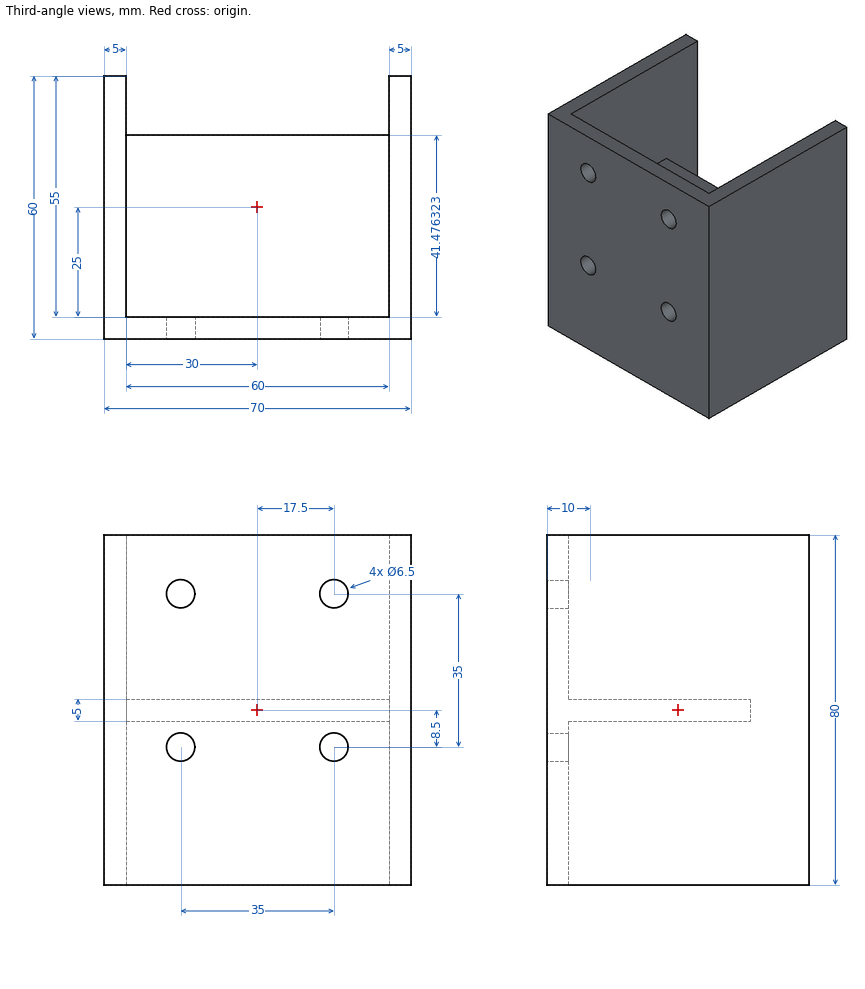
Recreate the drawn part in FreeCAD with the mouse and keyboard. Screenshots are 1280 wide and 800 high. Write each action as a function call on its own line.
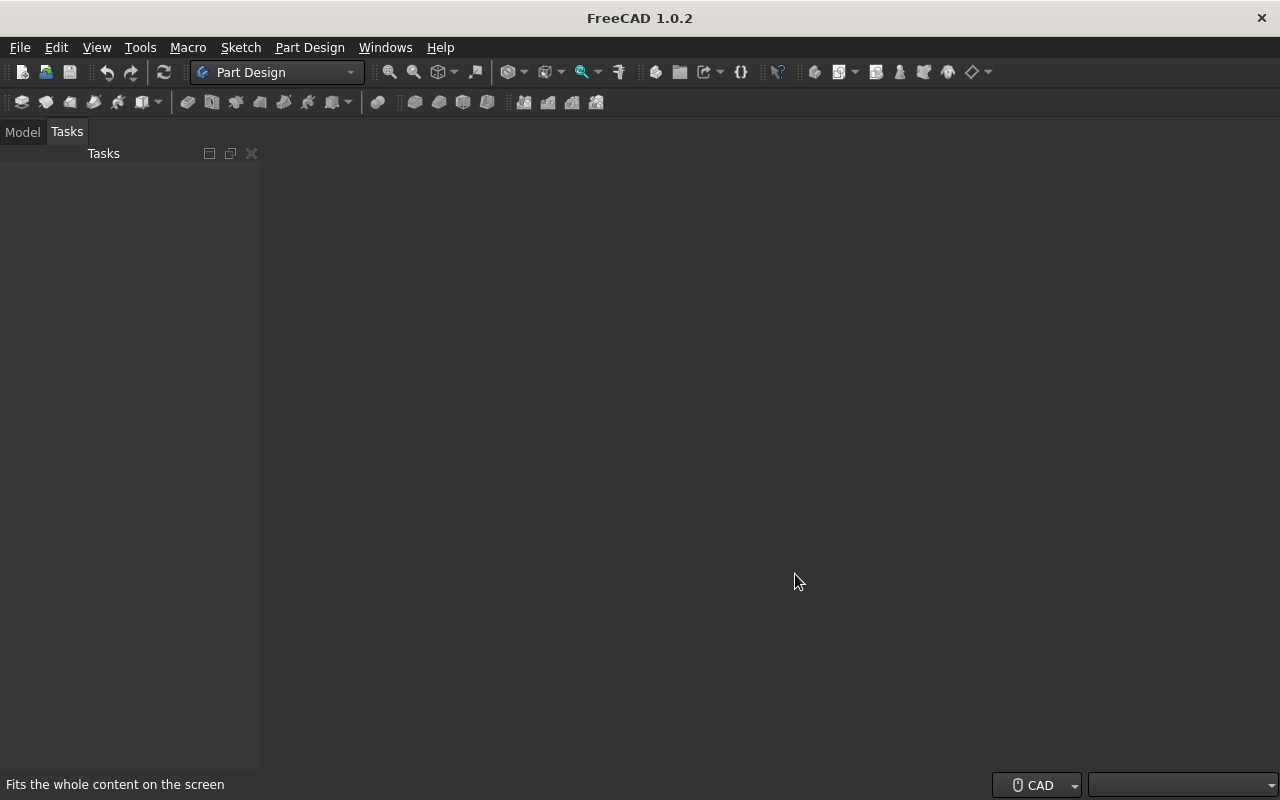
key(ctrl+n)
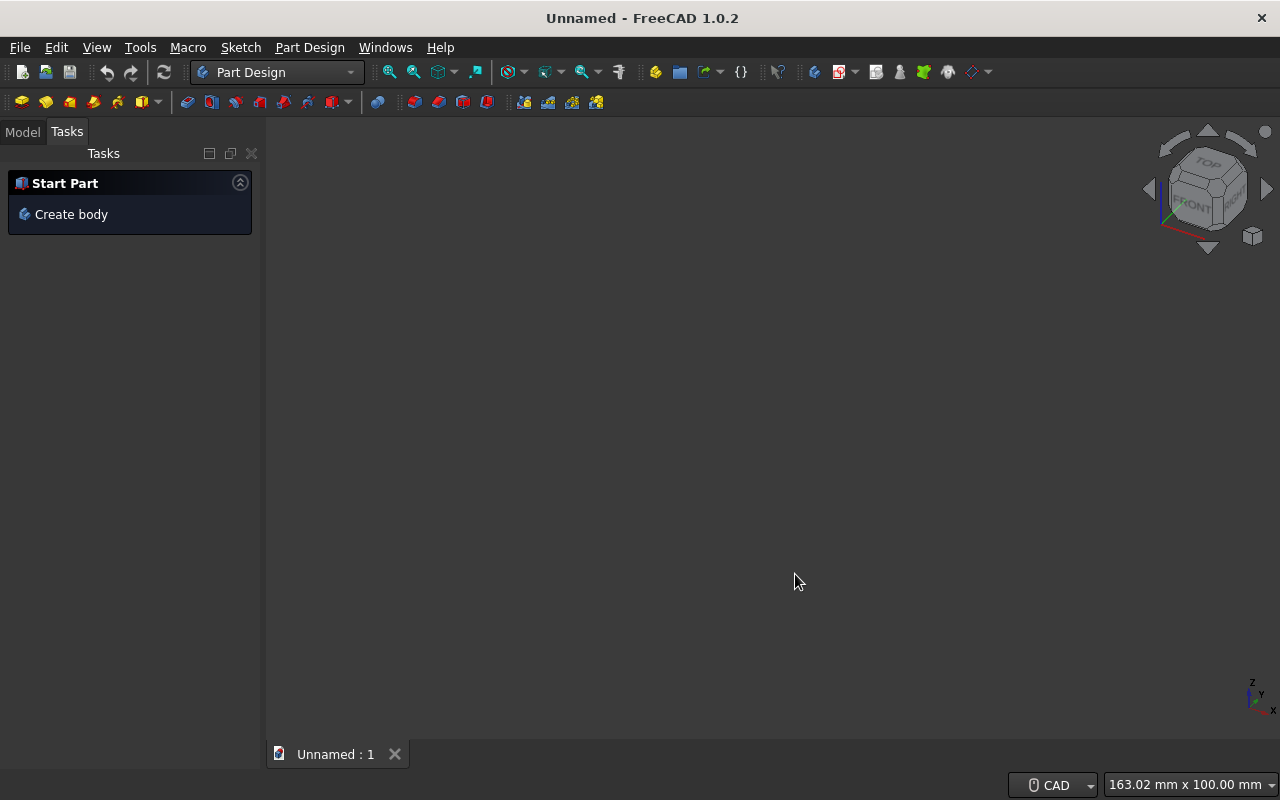
click(840, 72)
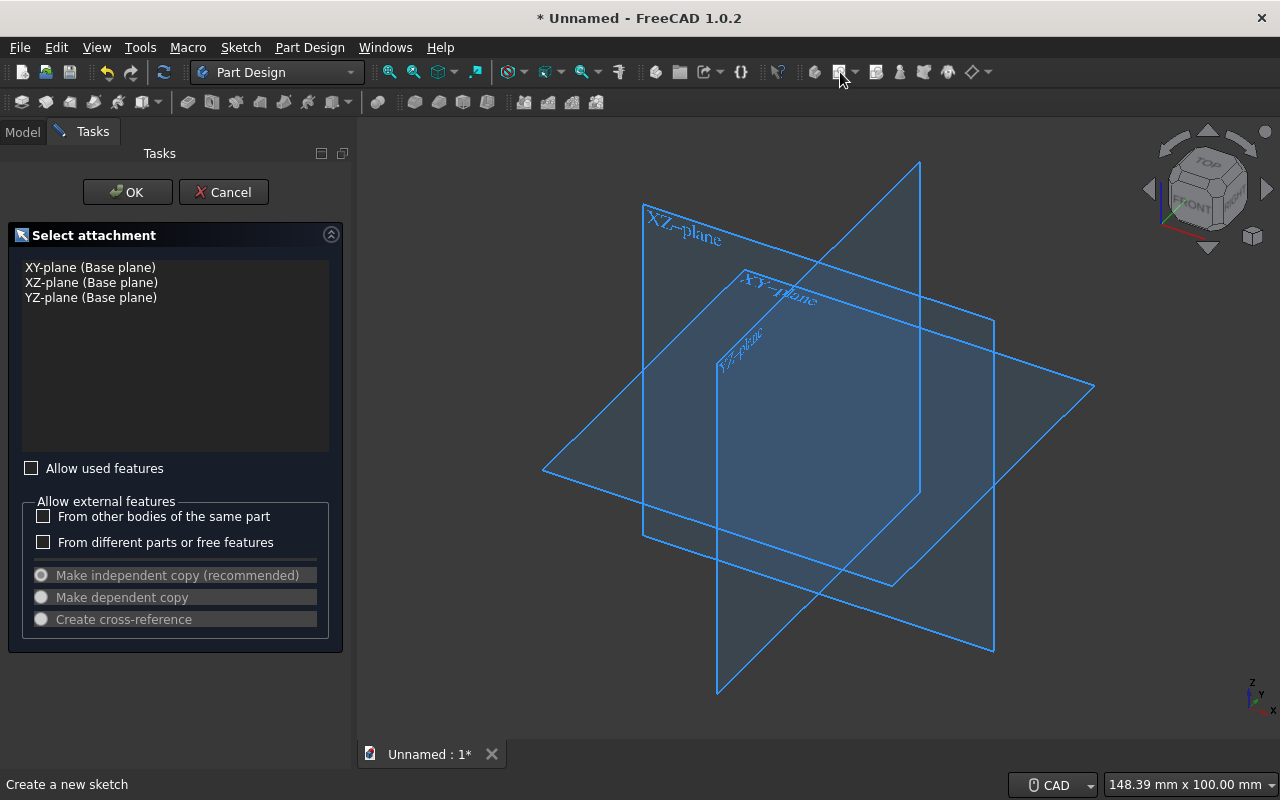
click(82, 268)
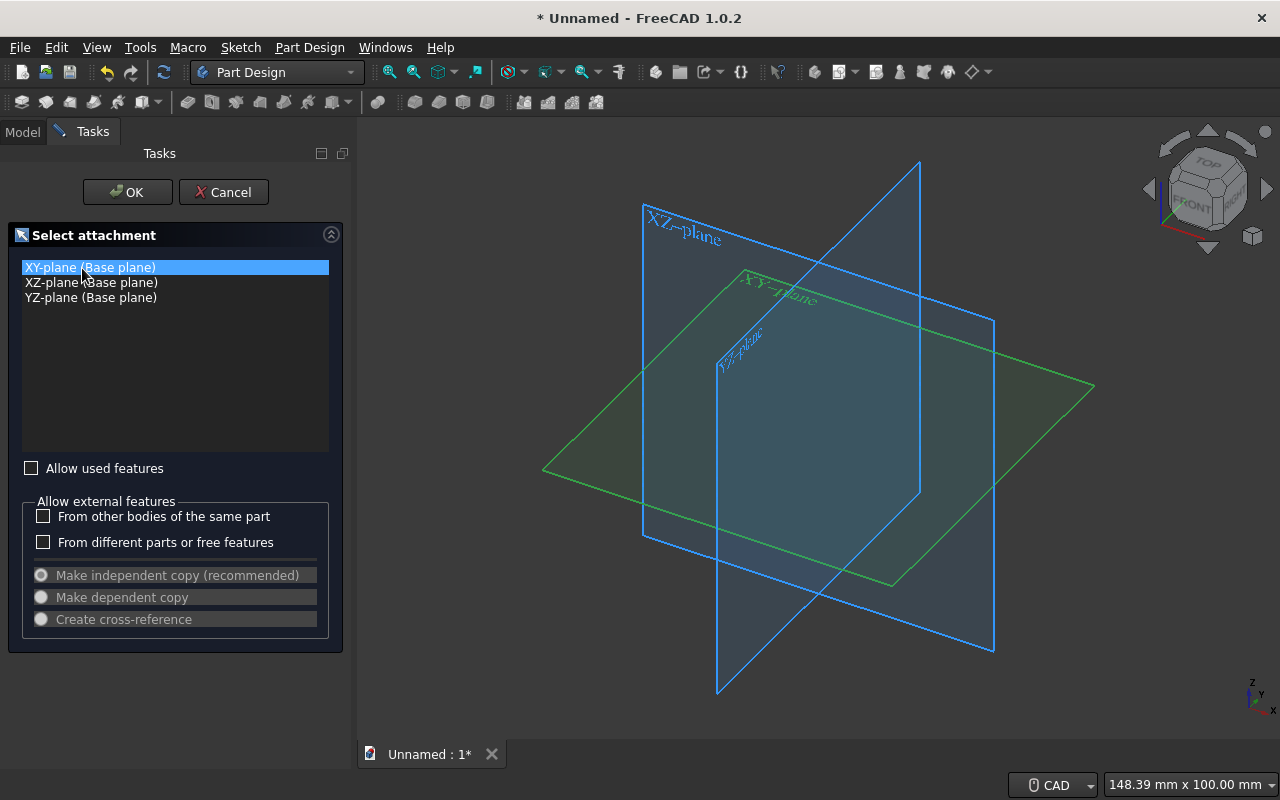
click(128, 192)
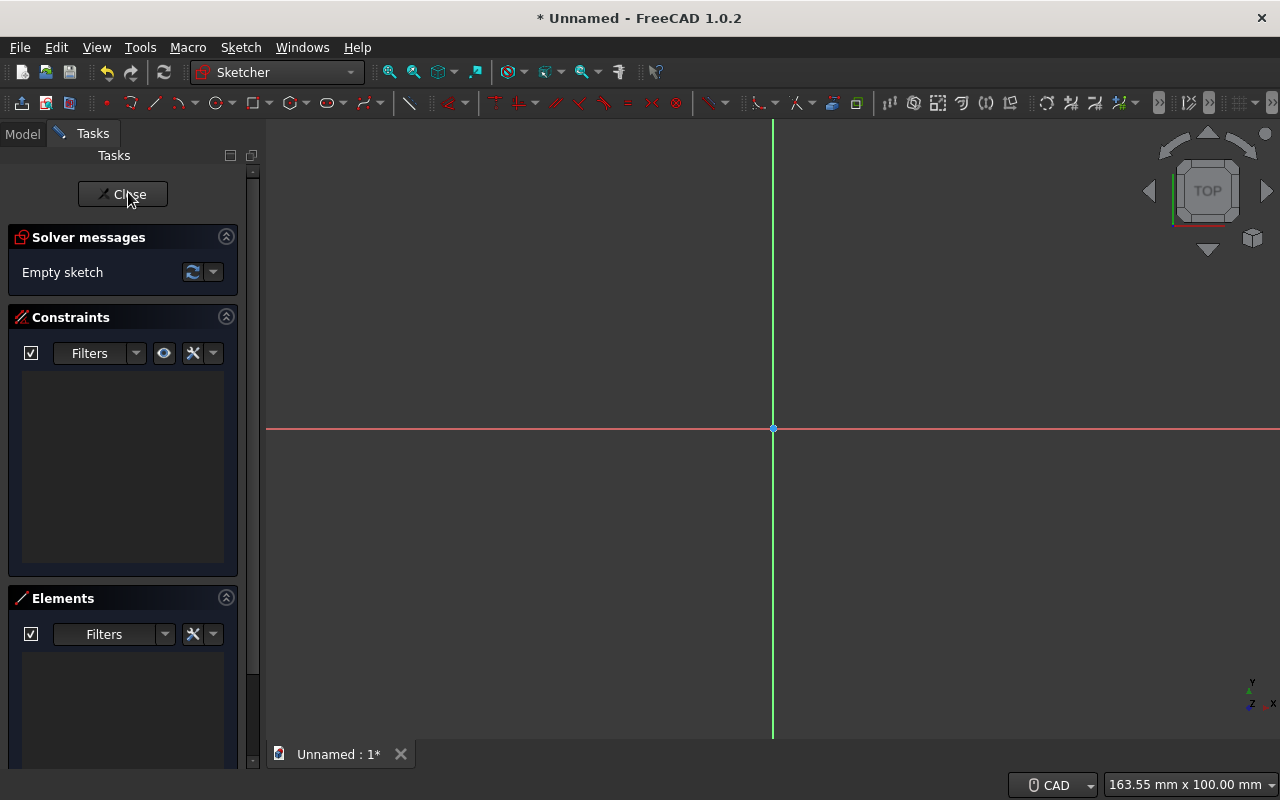
key(g)
key(m)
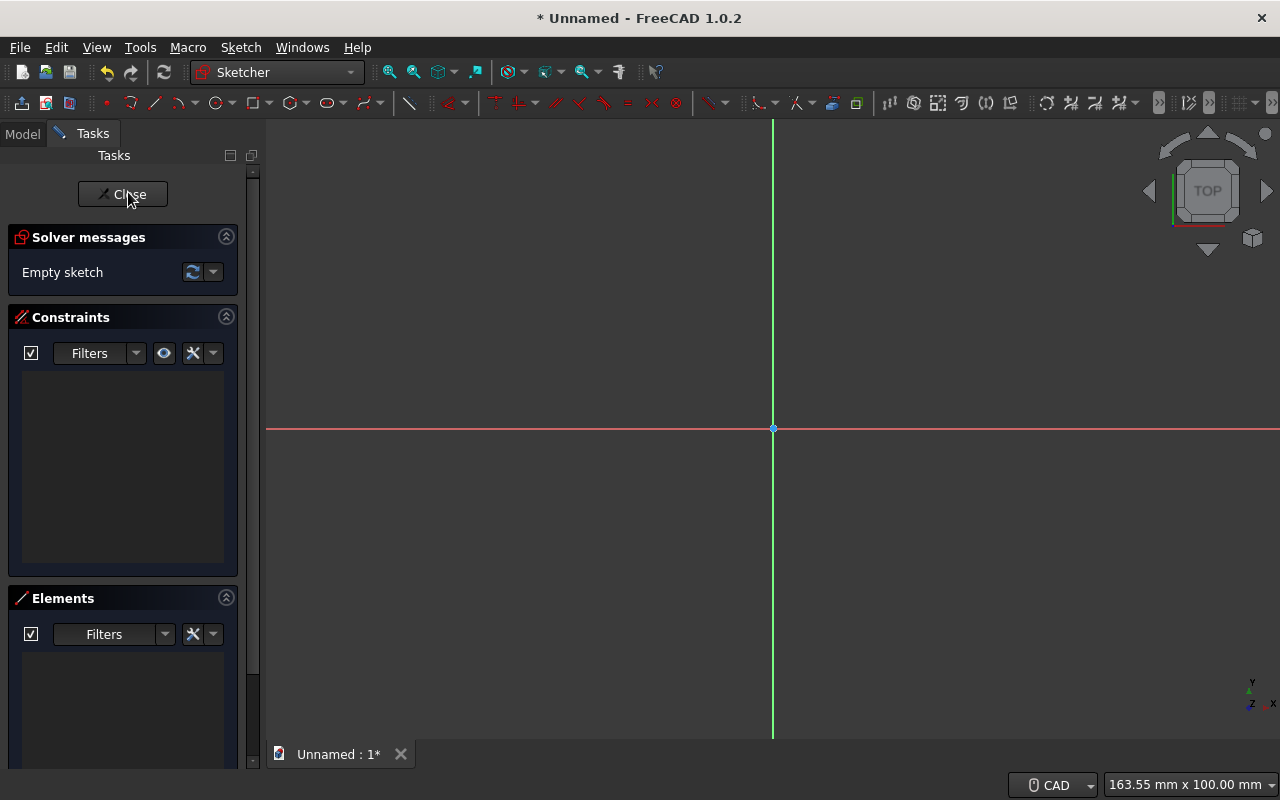
click(587, 584)
click(587, 243)
click(556, 243)
click(556, 615)
click(990, 615)
click(990, 243)
click(959, 243)
click(959, 584)
click(587, 585)
key(Escape)
key(Escape)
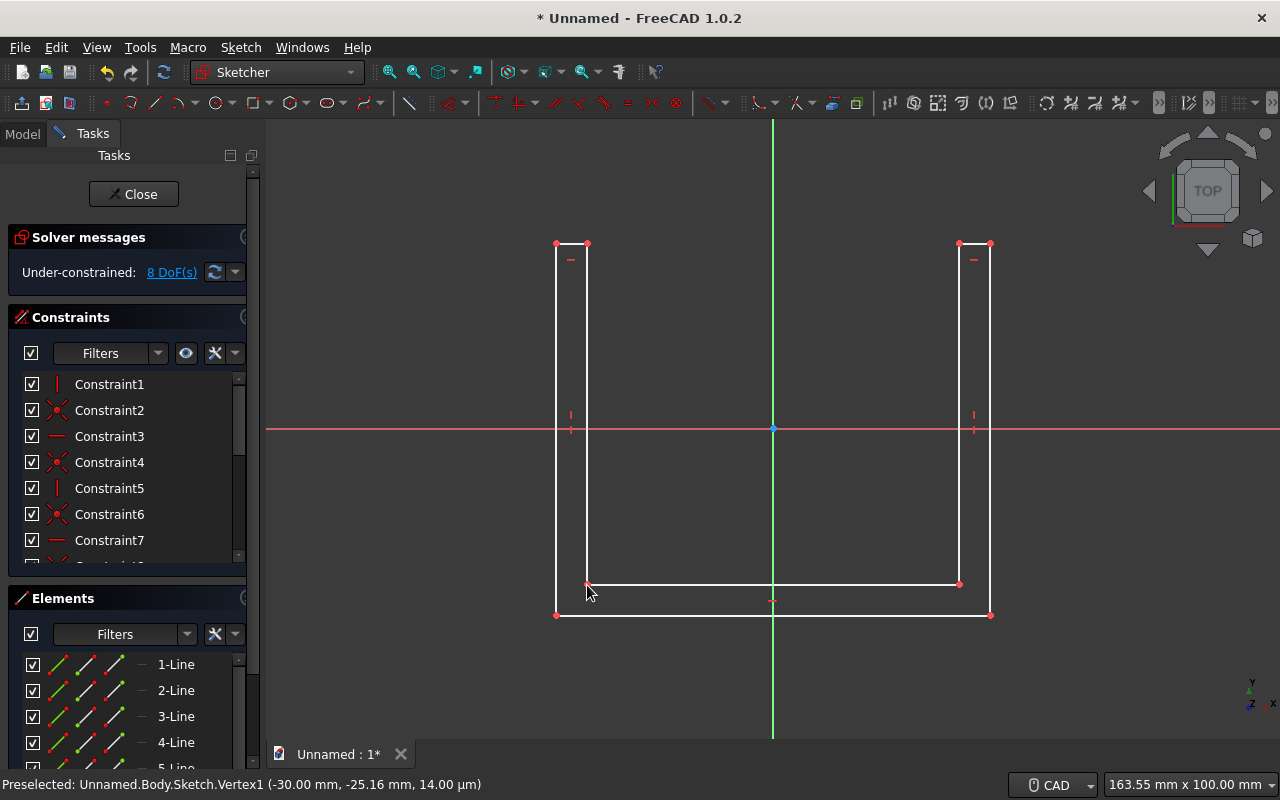
scroll(578, 244, up, 2)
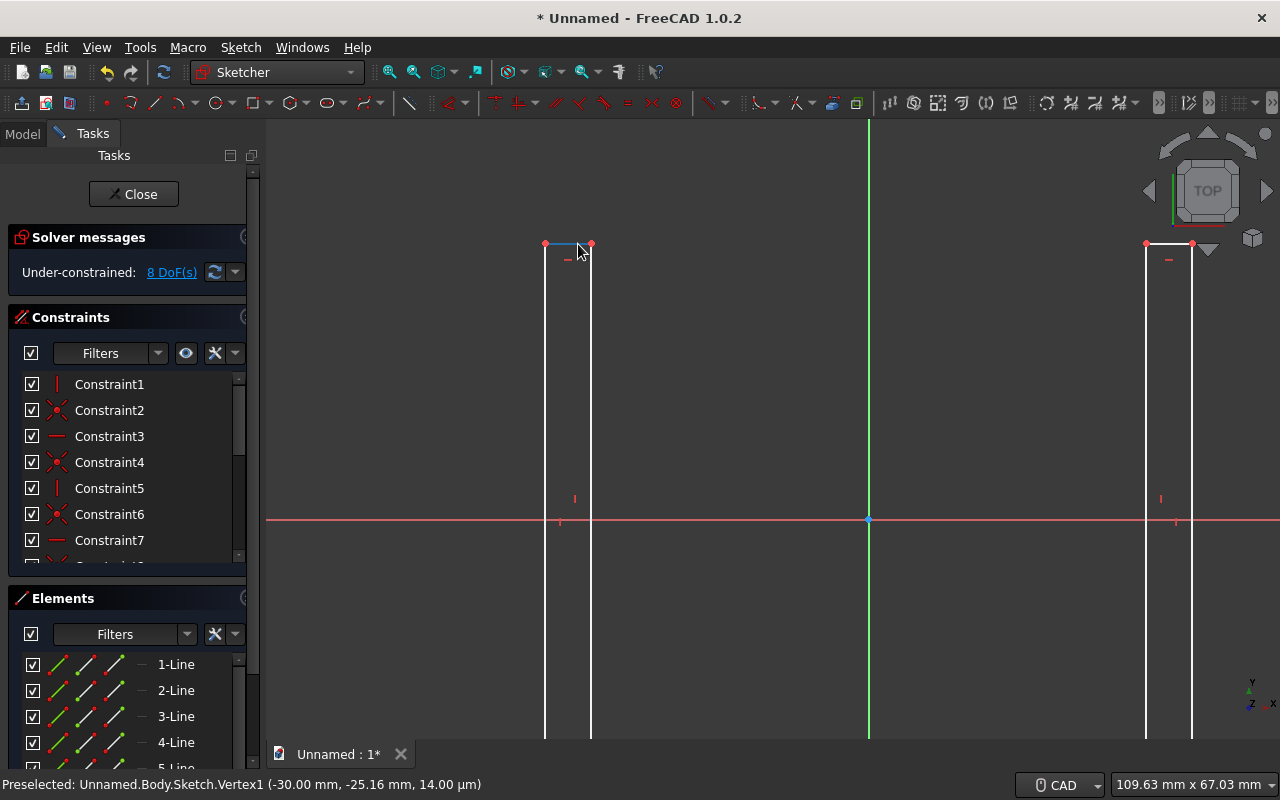
click(577, 244)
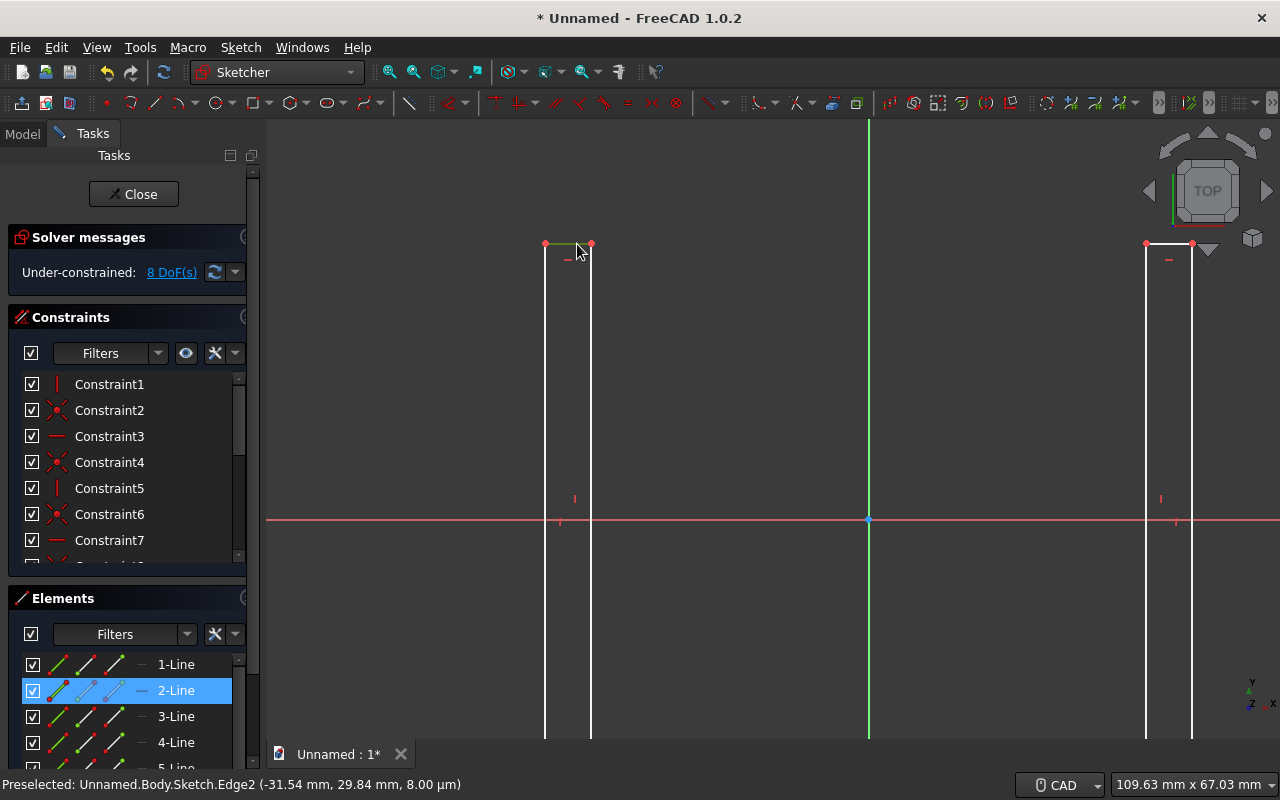
key(l)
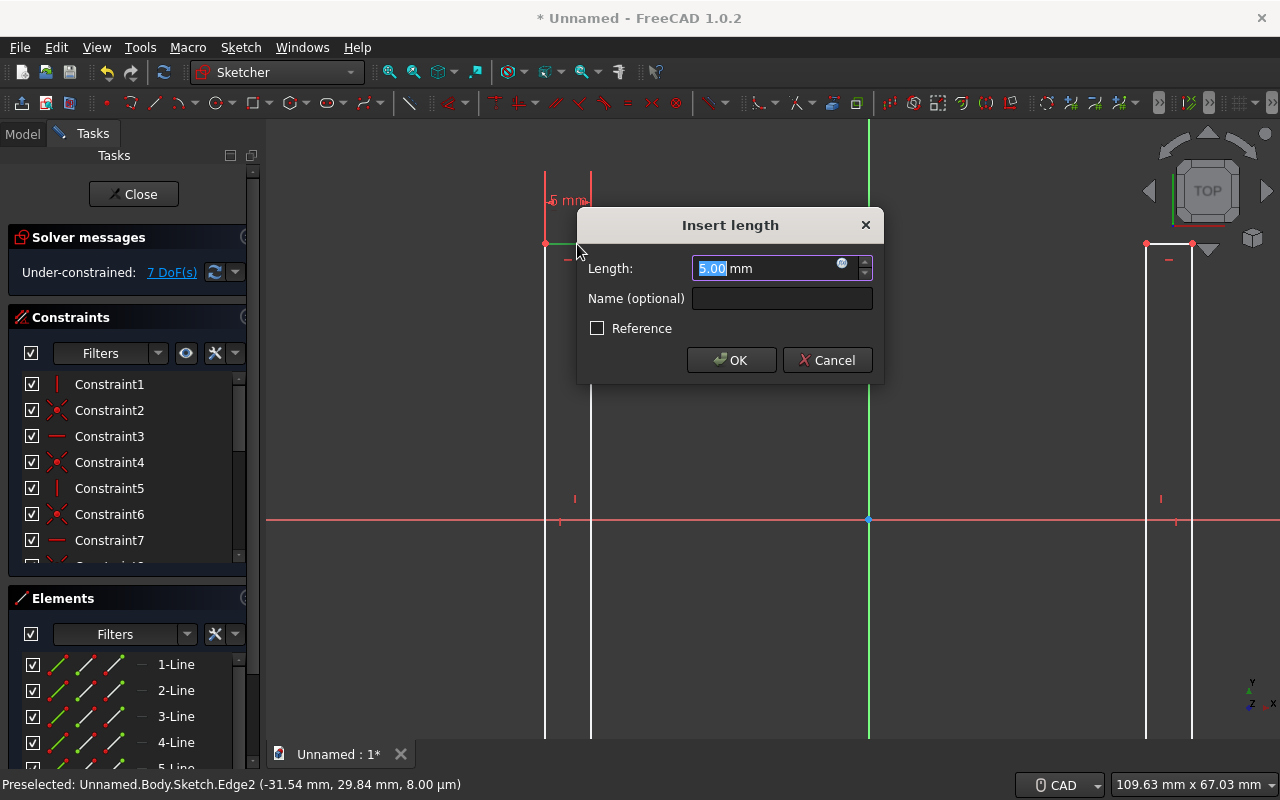
text(5)
key(Return)